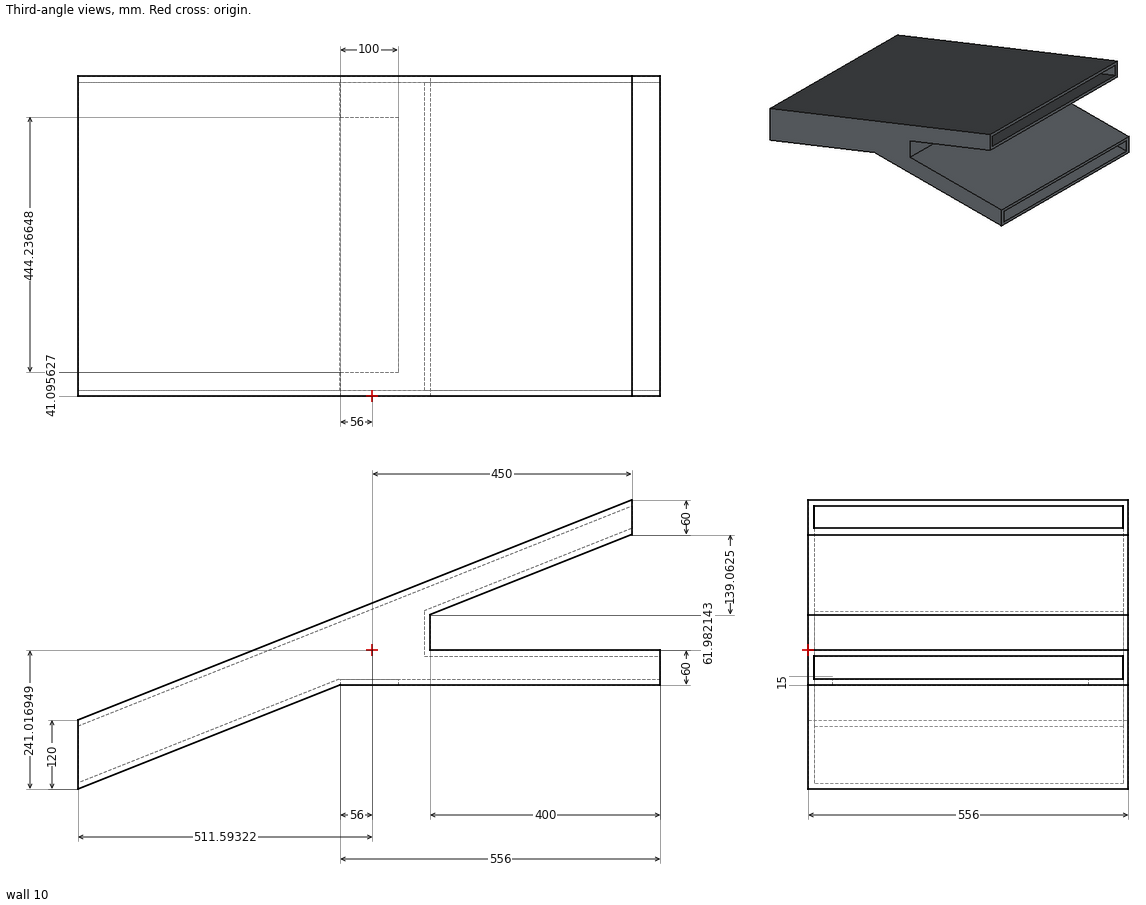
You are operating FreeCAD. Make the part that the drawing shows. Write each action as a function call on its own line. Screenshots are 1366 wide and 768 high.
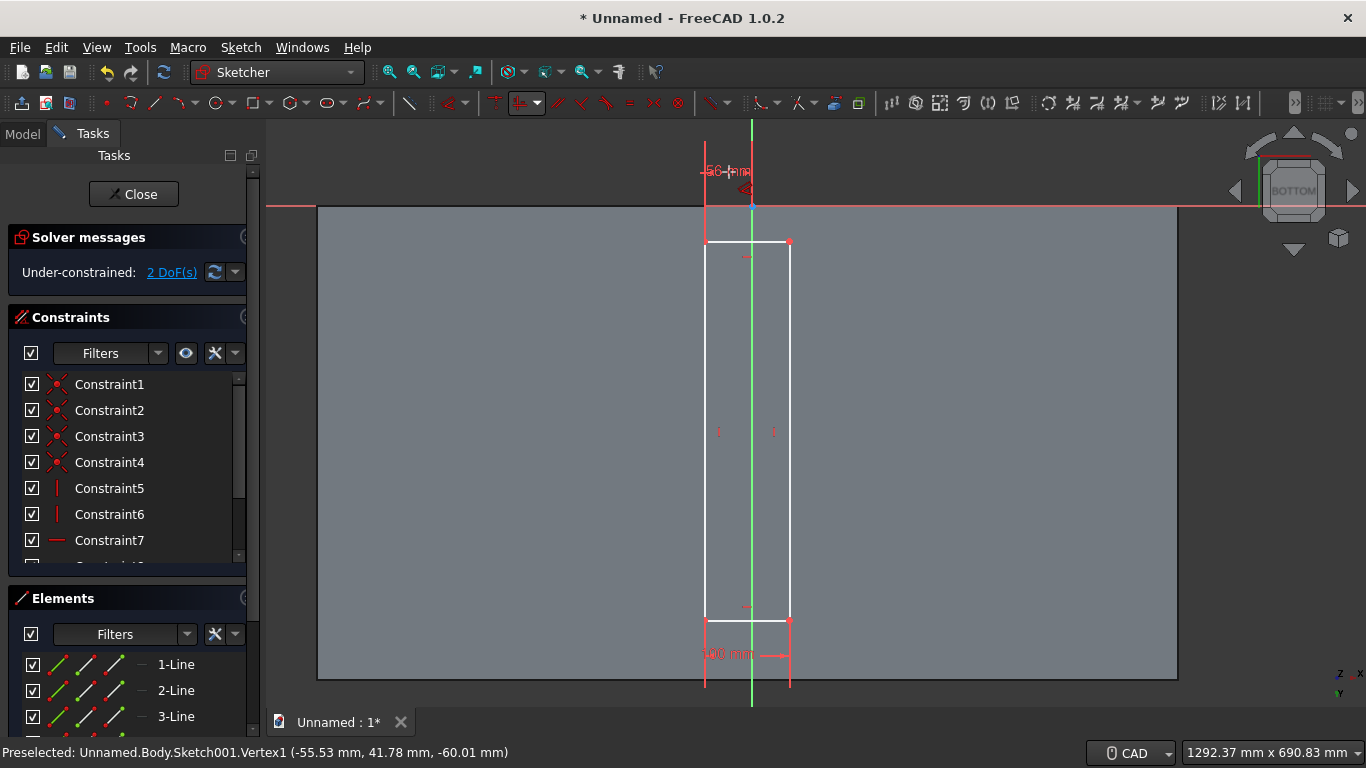
click(705, 356)
click(671, 432)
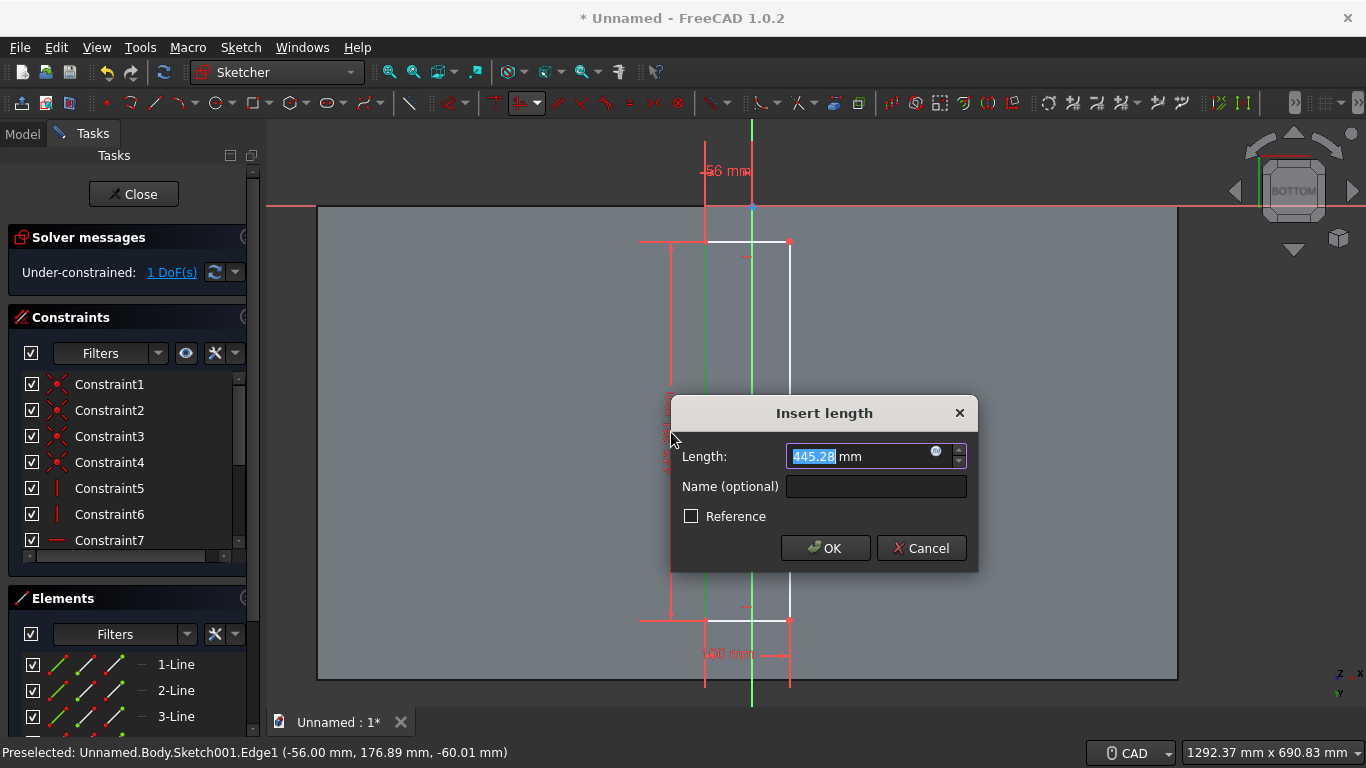
text(444.236648)
key(Return)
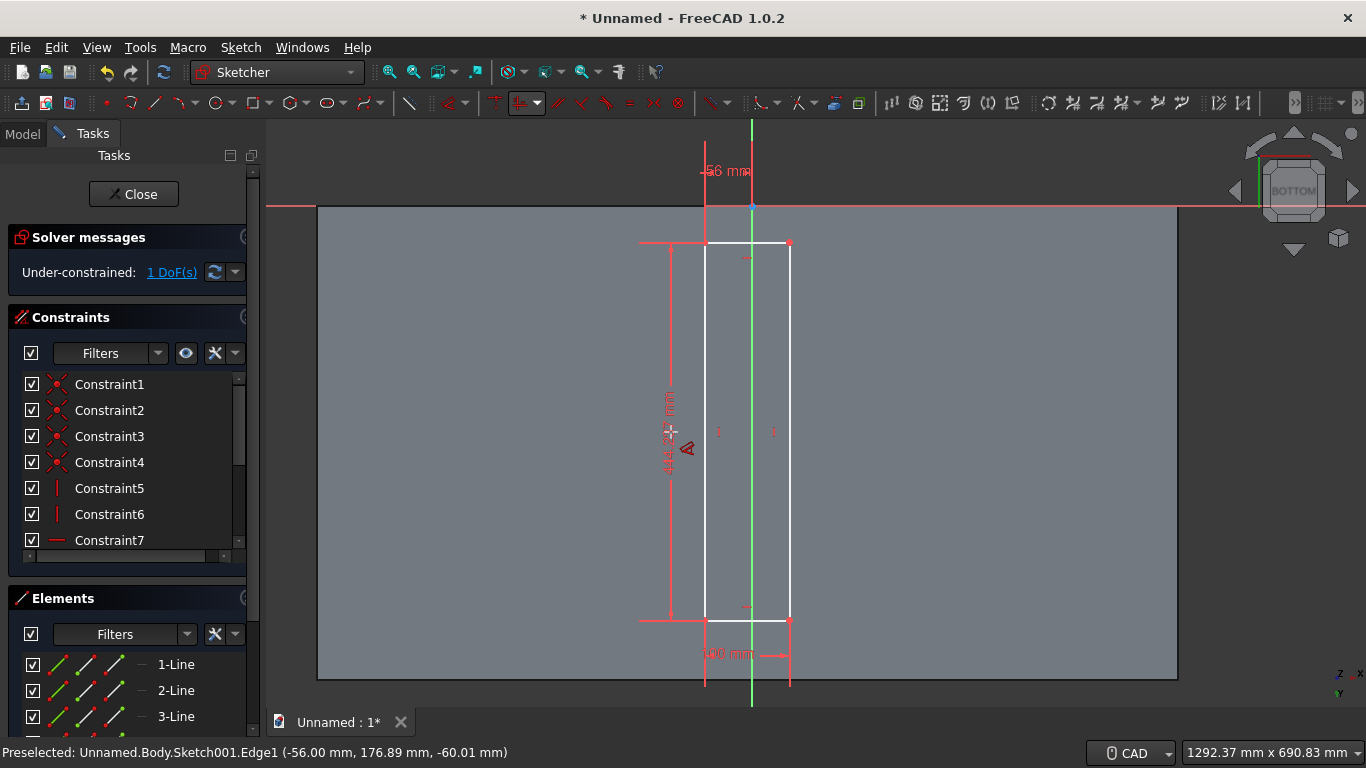
click(705, 243)
click(671, 225)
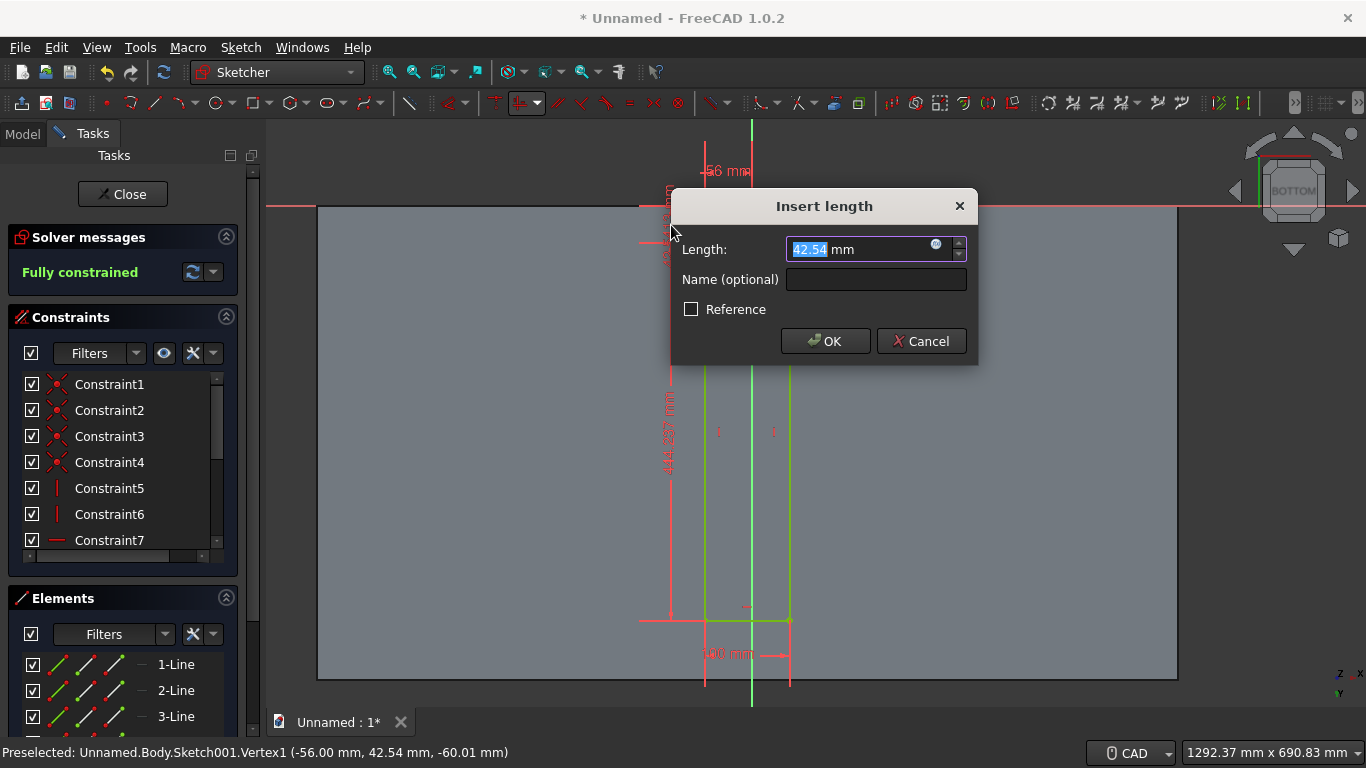
text(41.095627)
key(Return)
key(Escape)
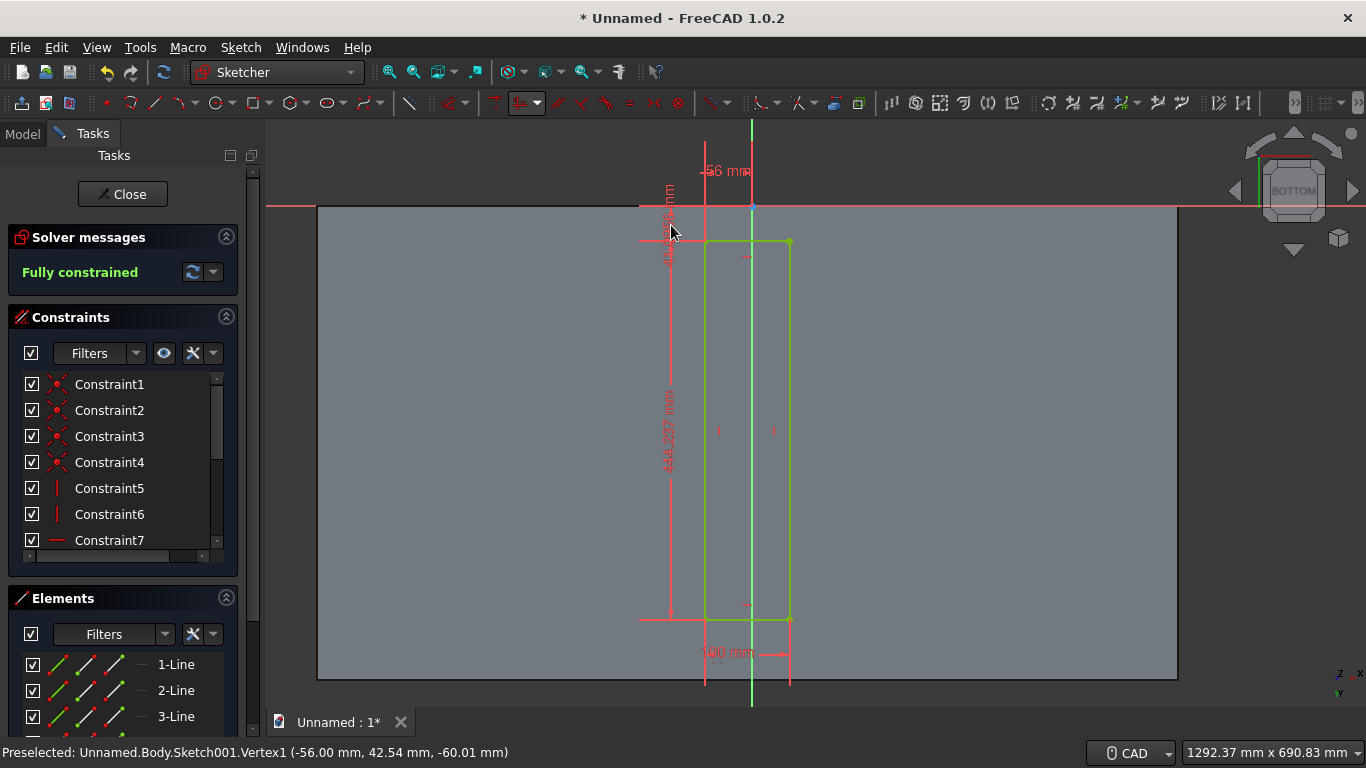
click(123, 194)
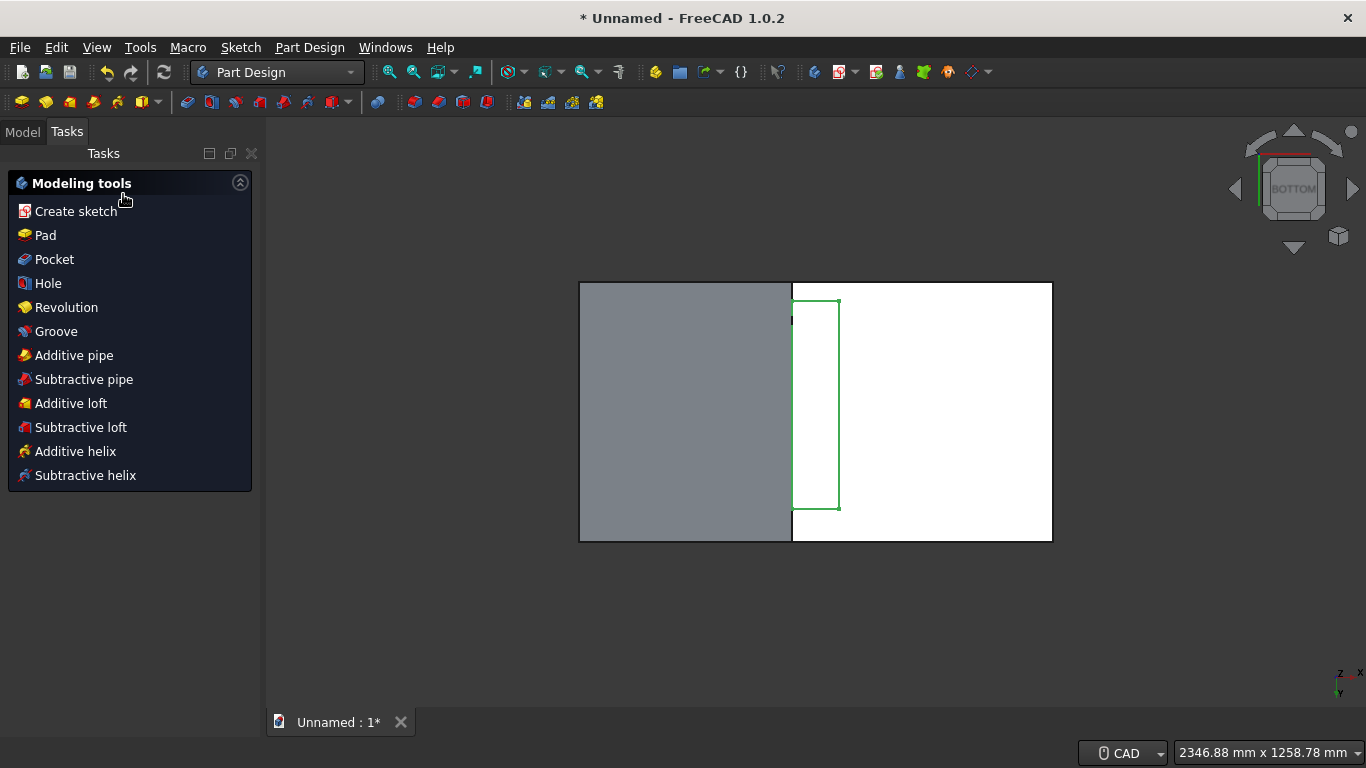
click(188, 102)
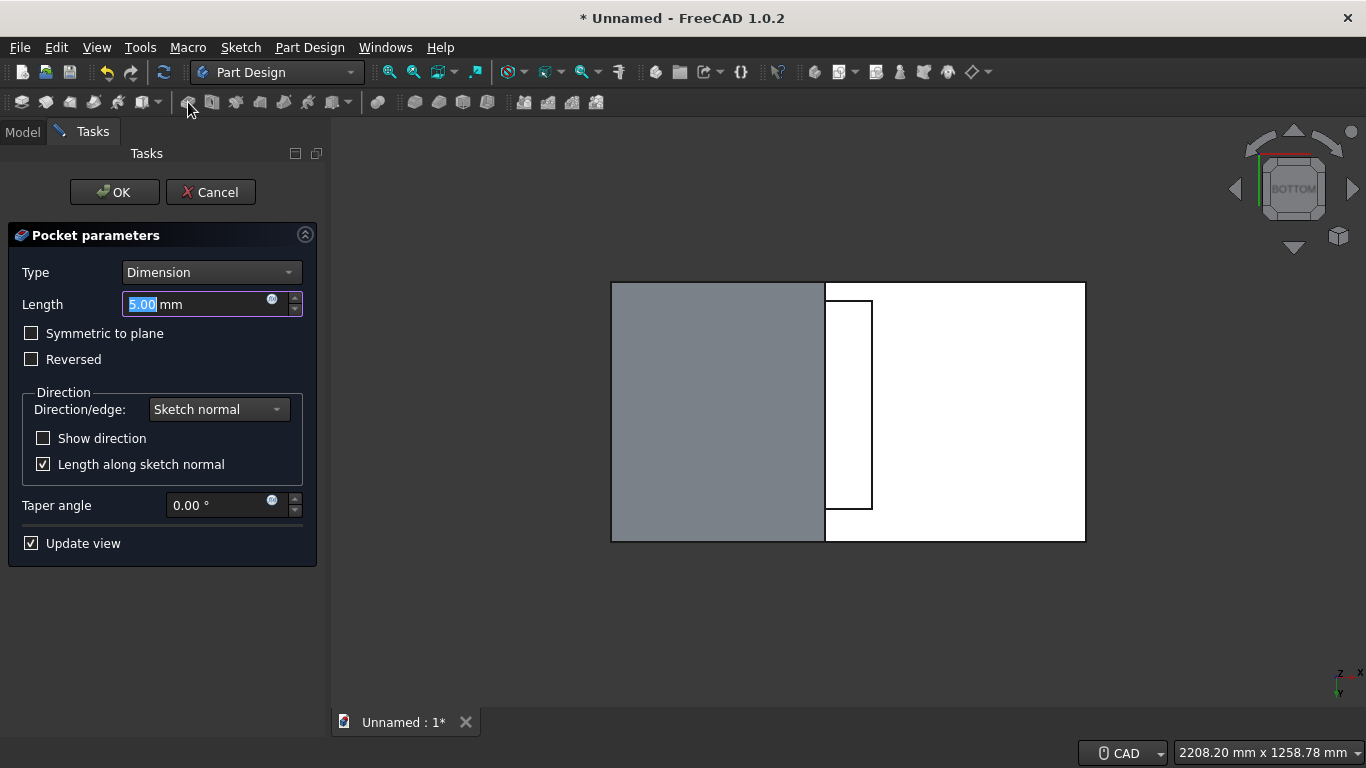
text(15)
key(Tab)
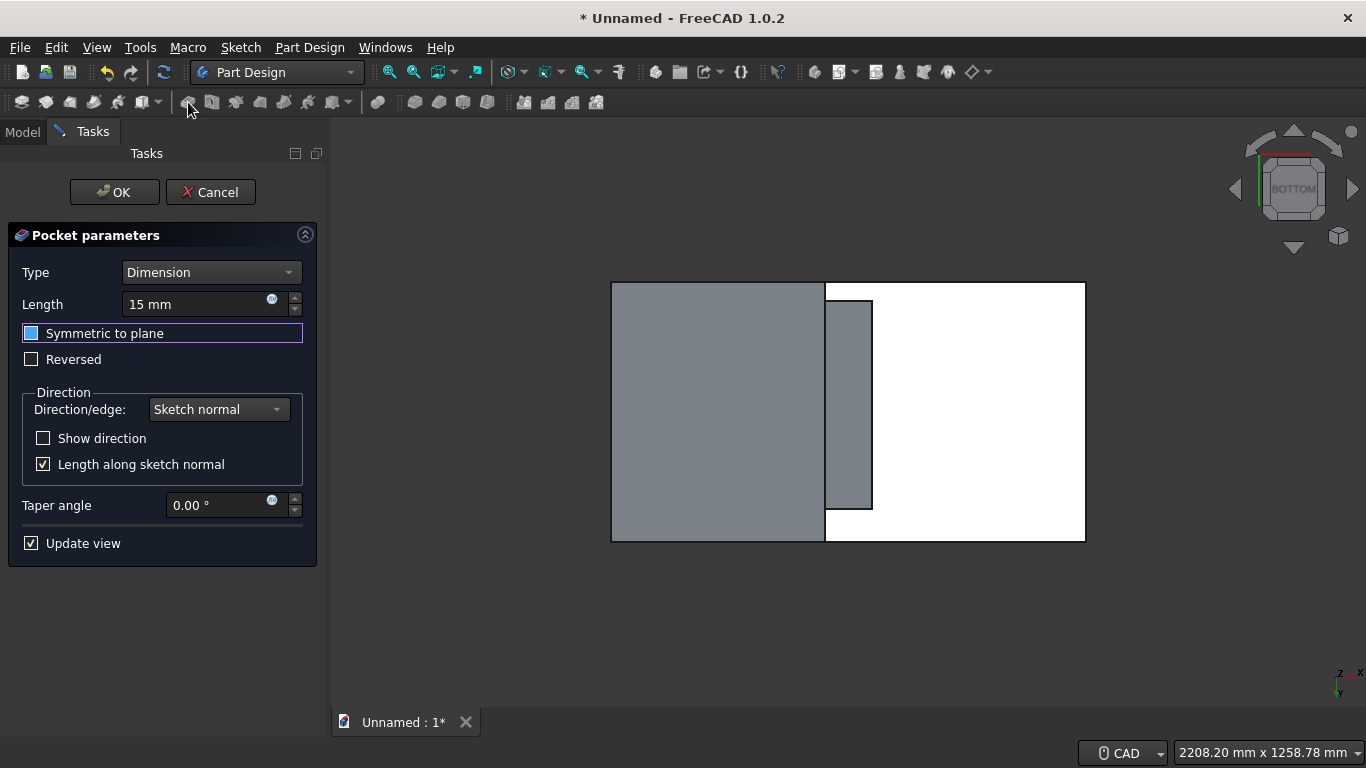
click(115, 192)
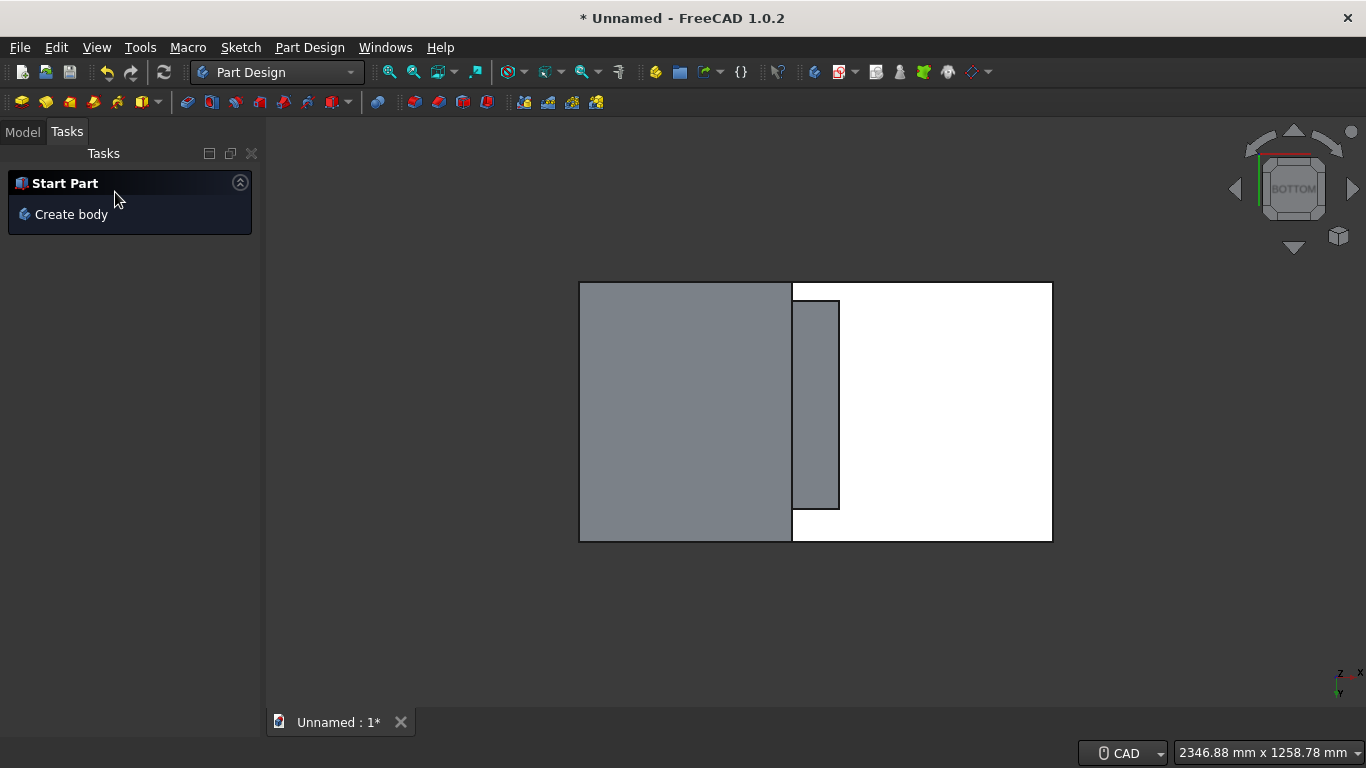
key(0)